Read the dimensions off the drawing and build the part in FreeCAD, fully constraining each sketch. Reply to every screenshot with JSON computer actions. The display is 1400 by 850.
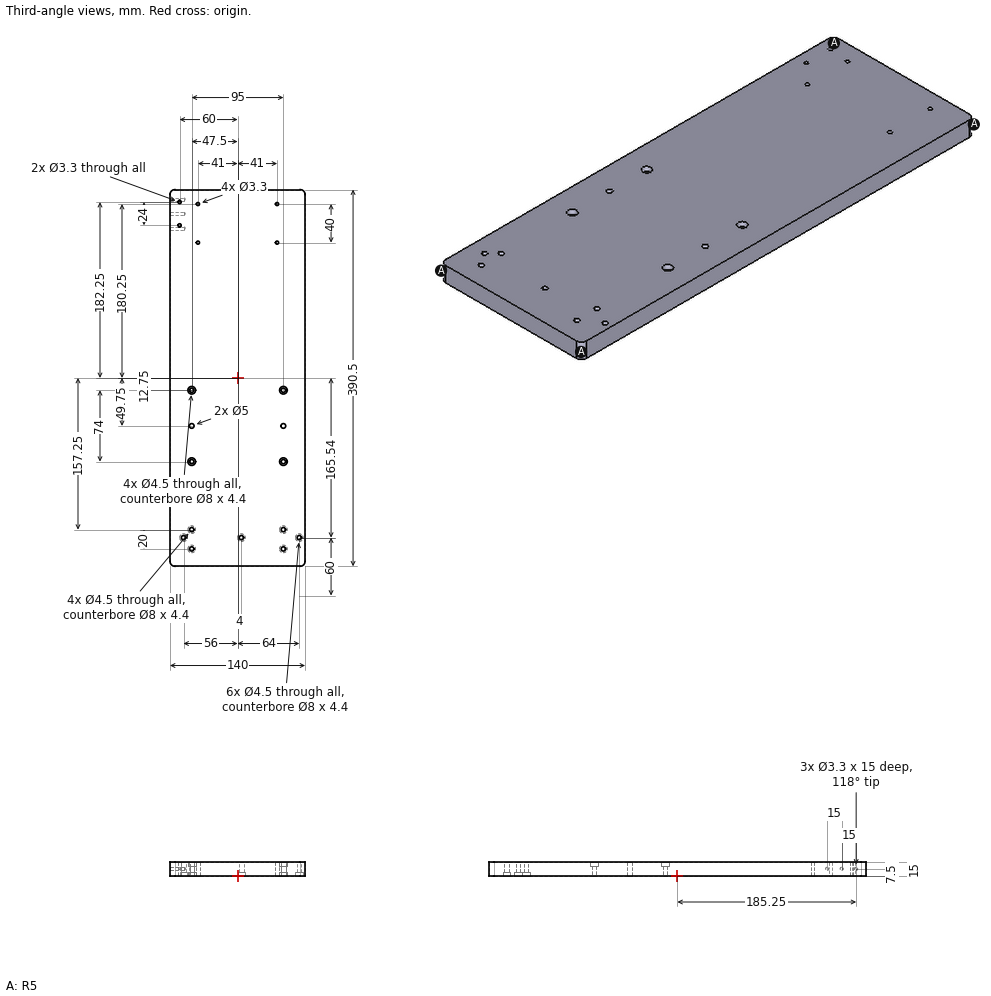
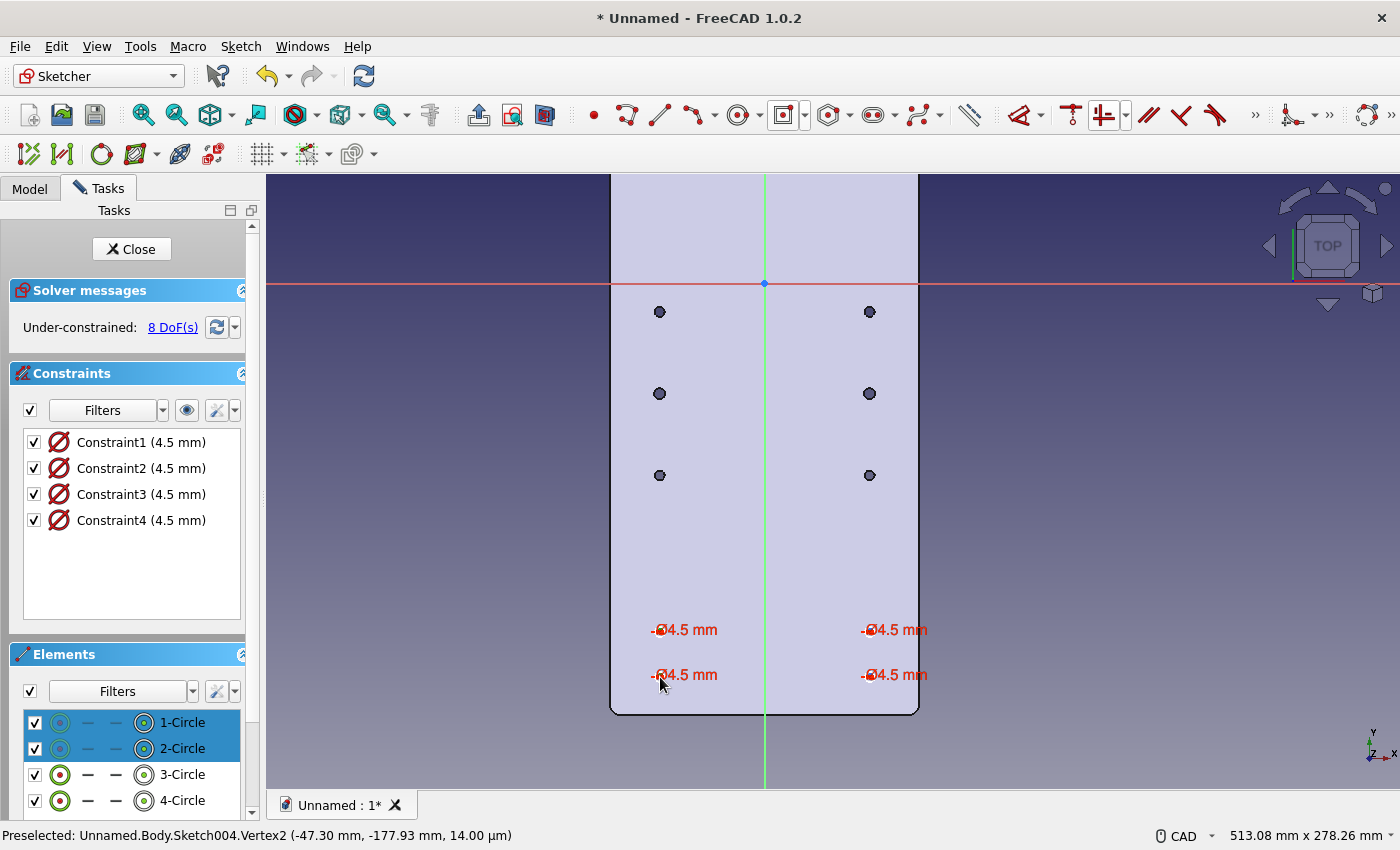
{"action": "key", "text": "v"}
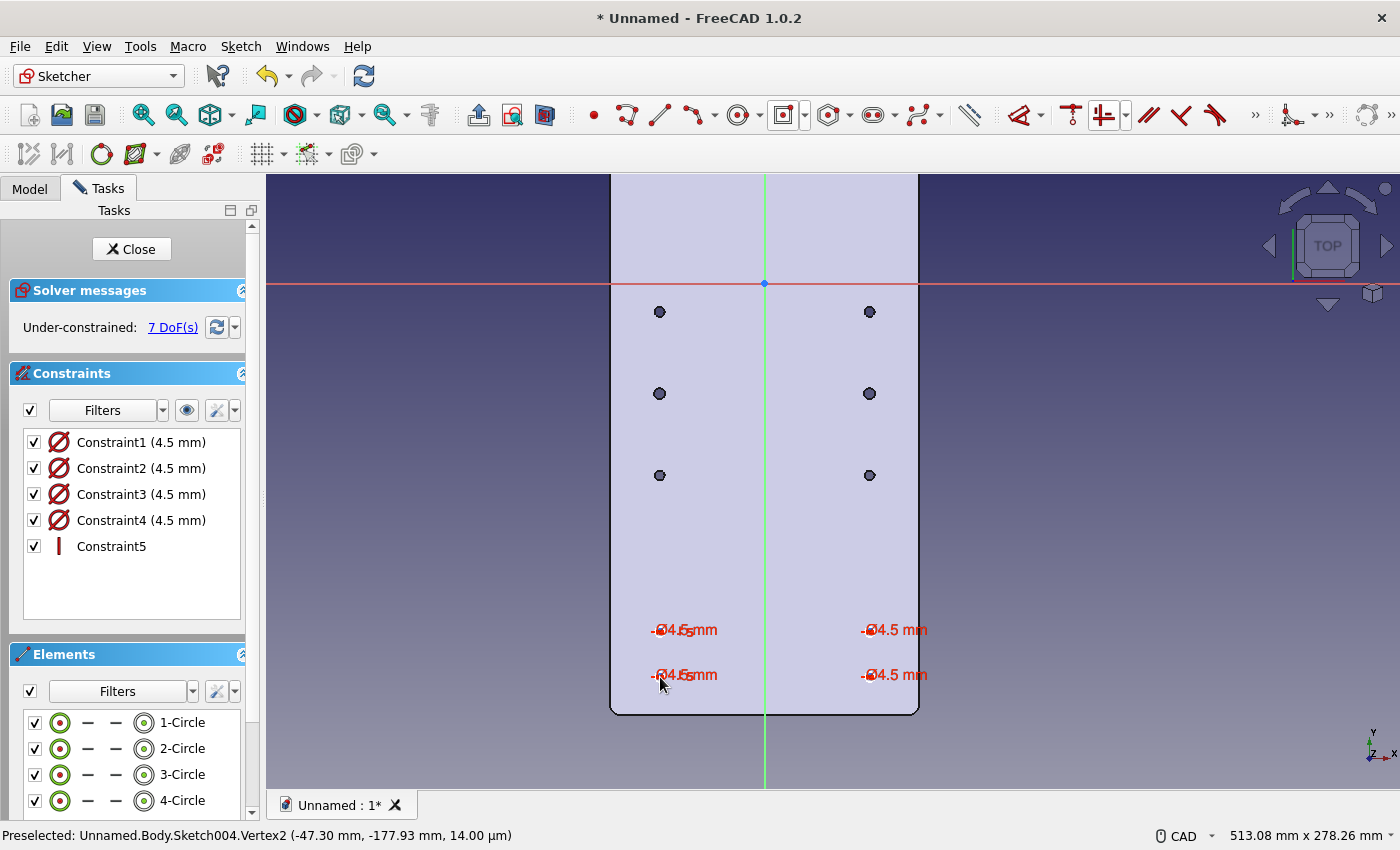
{"action": "left_click", "coordinate": [660, 632]}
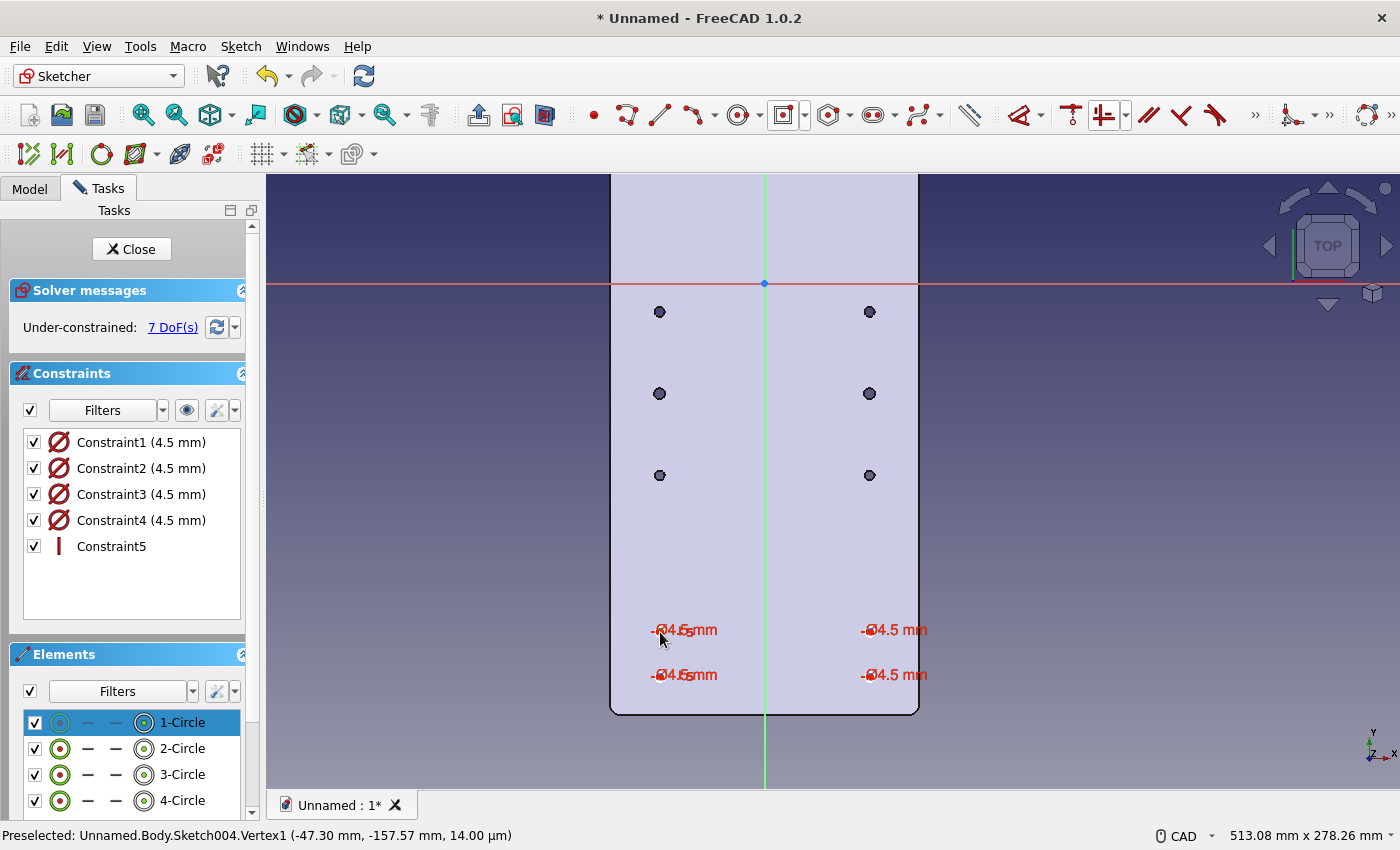
{"action": "left_click", "coordinate": [870, 632]}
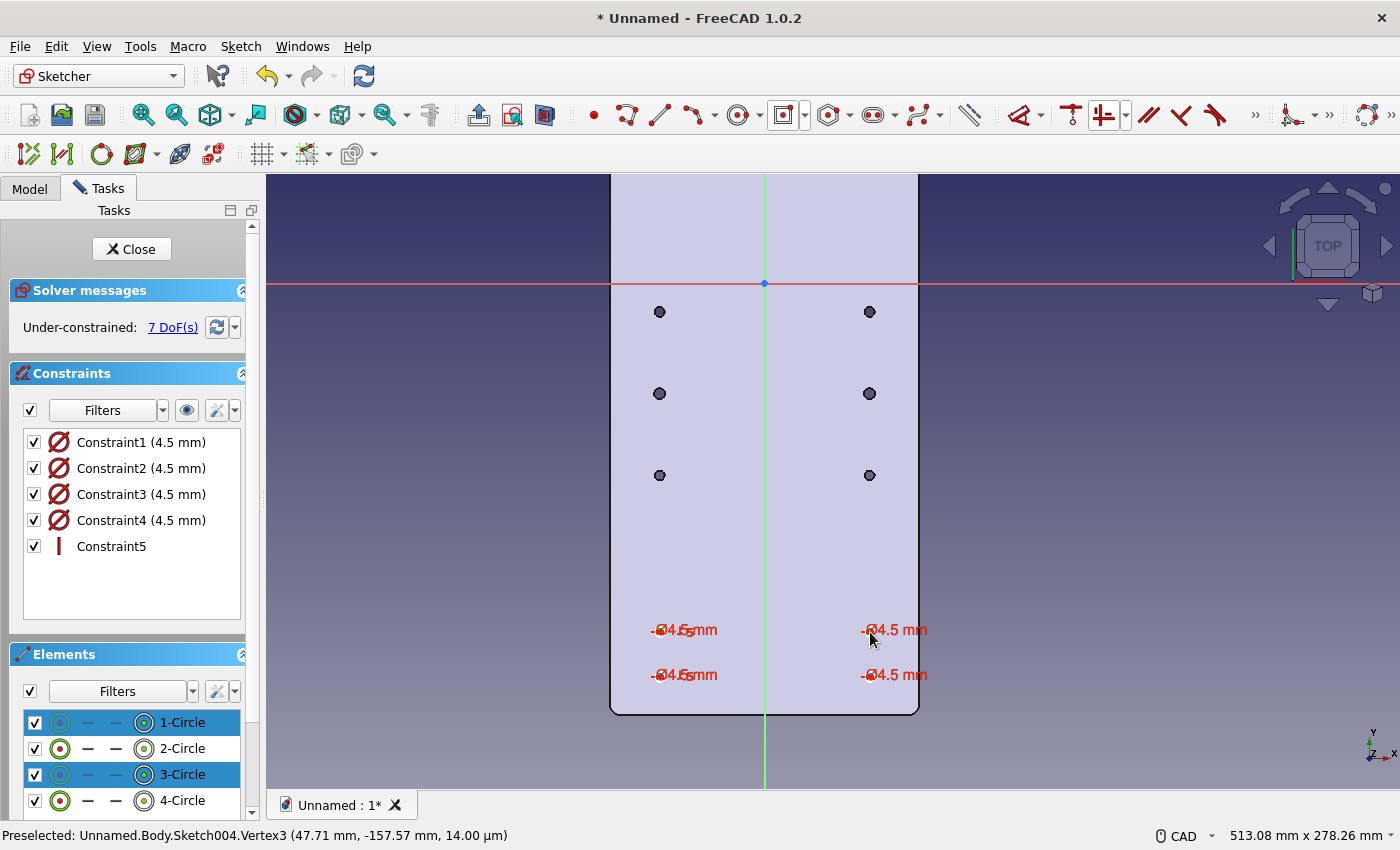
{"action": "key", "text": "h"}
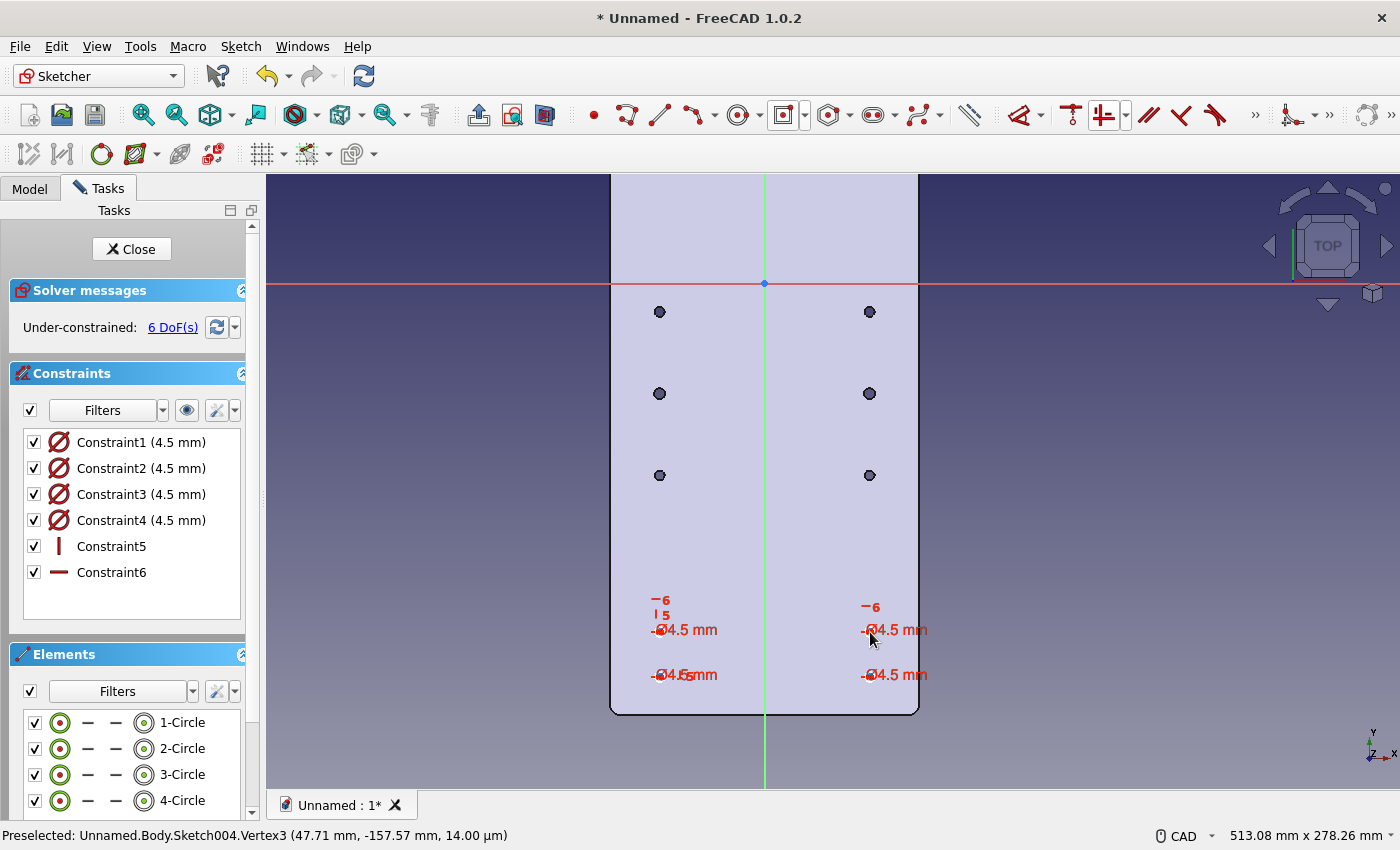
{"action": "left_click", "coordinate": [870, 632]}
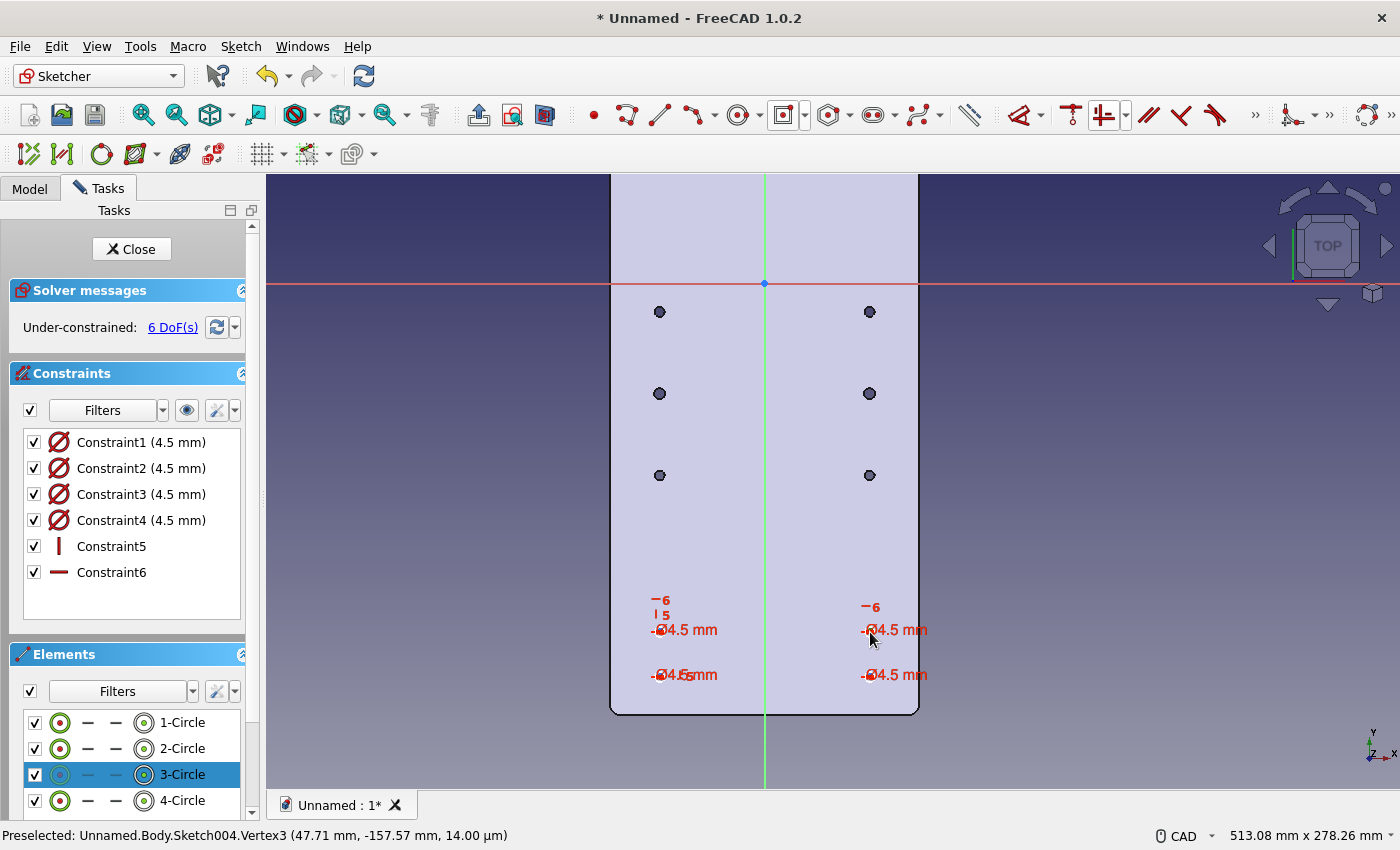
{"action": "left_click", "coordinate": [870, 677]}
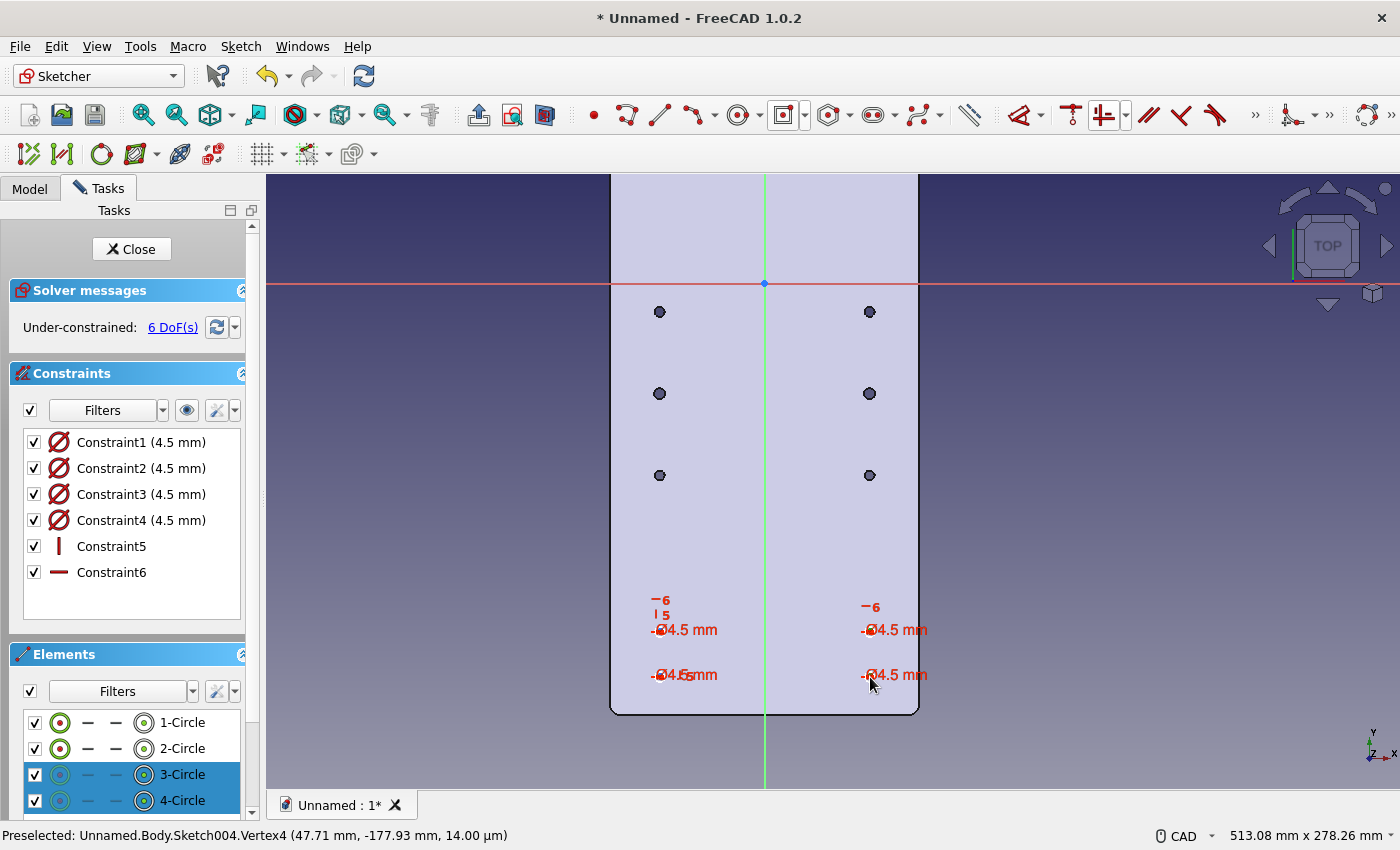
{"action": "left_click", "coordinate": [1126, 116]}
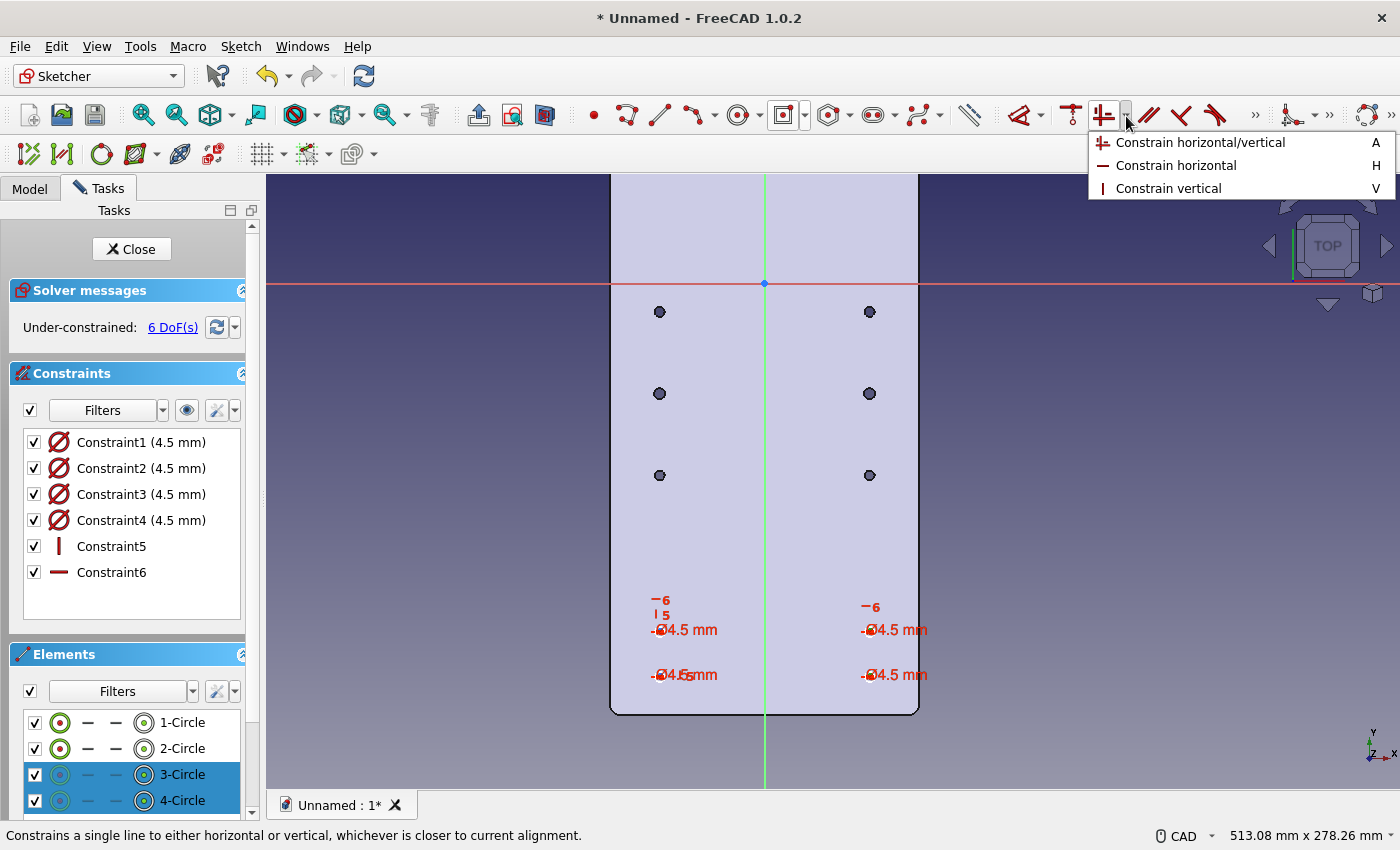
{"action": "left_click", "coordinate": [1242, 188]}